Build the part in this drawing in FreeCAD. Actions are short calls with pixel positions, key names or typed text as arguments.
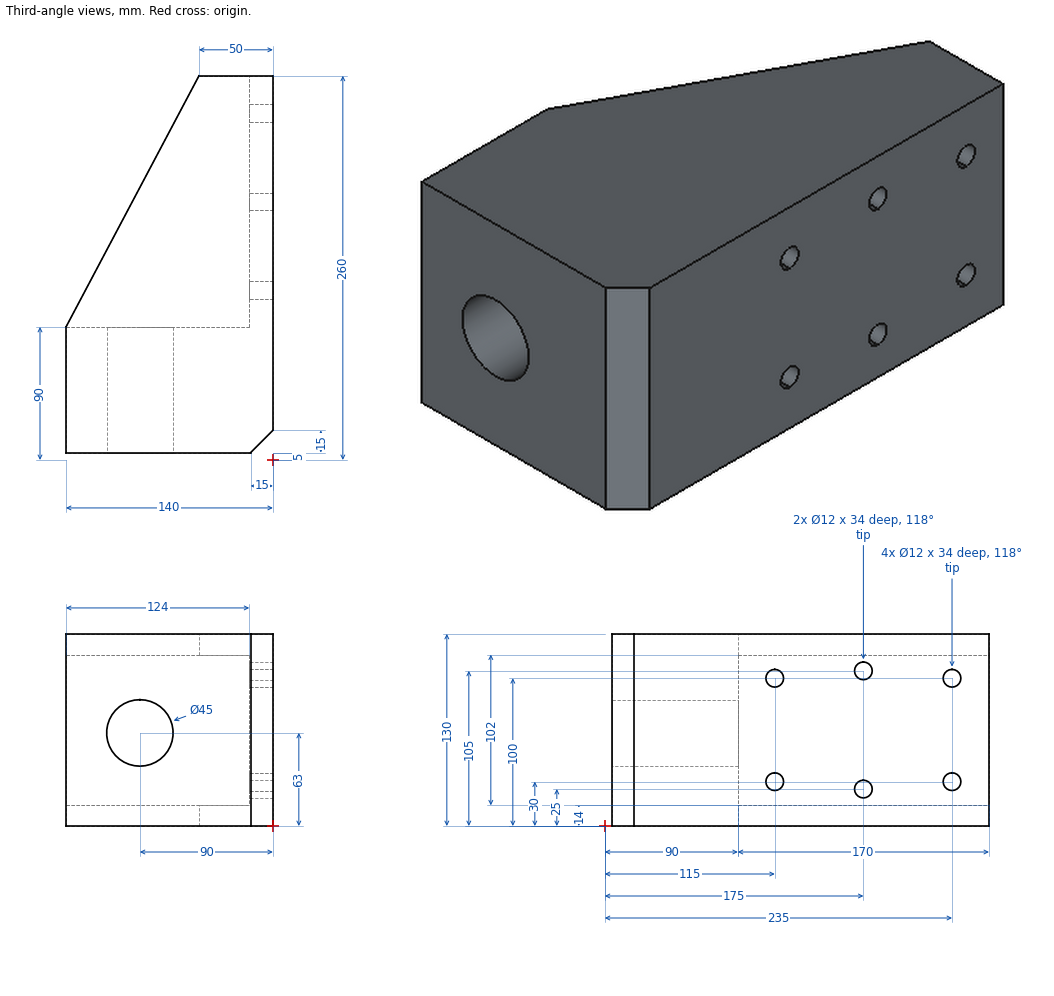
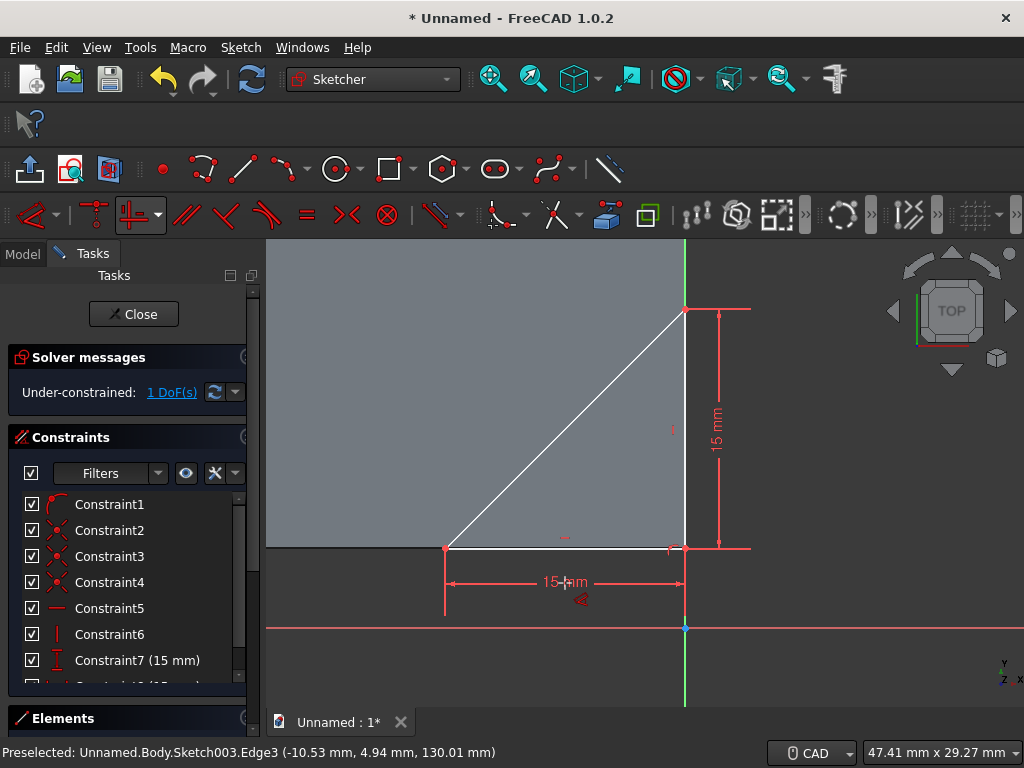
click(685, 549)
click(719, 589)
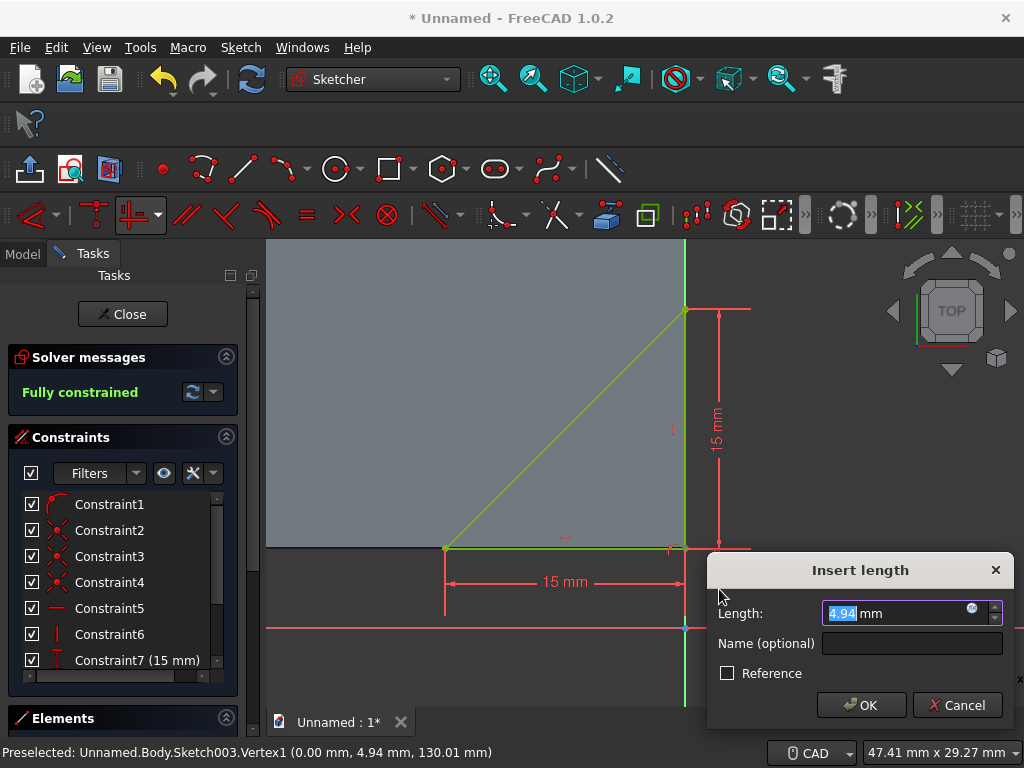
text(5)
key(Return)
key(Escape)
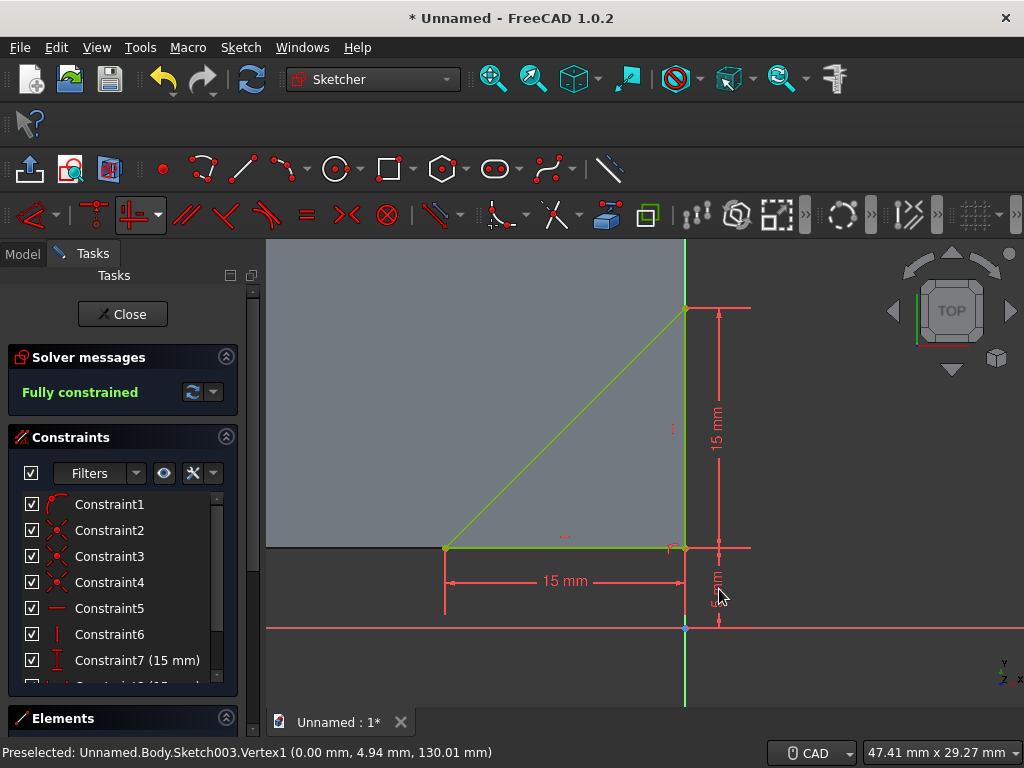
click(123, 314)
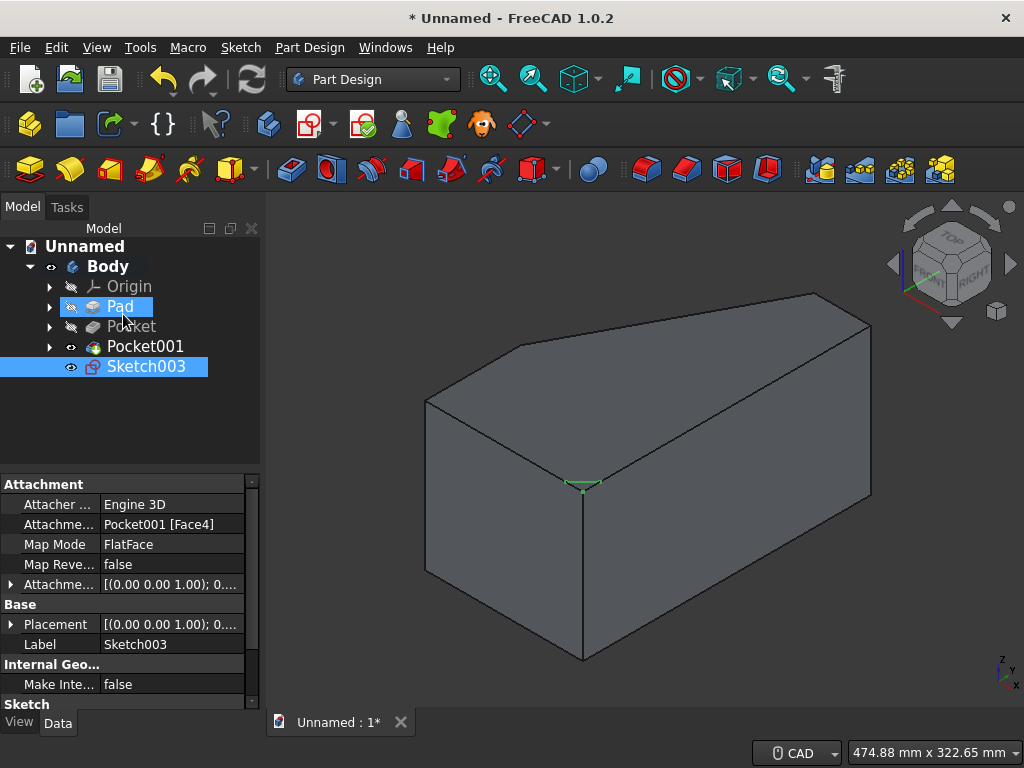
click(292, 170)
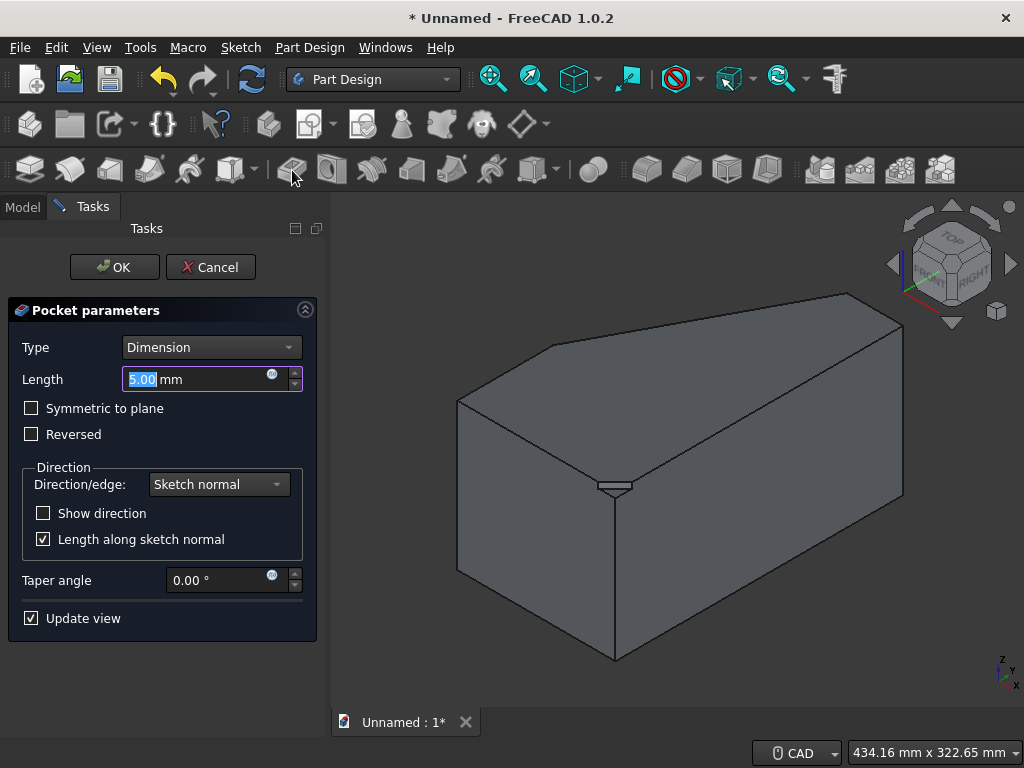
click(212, 348)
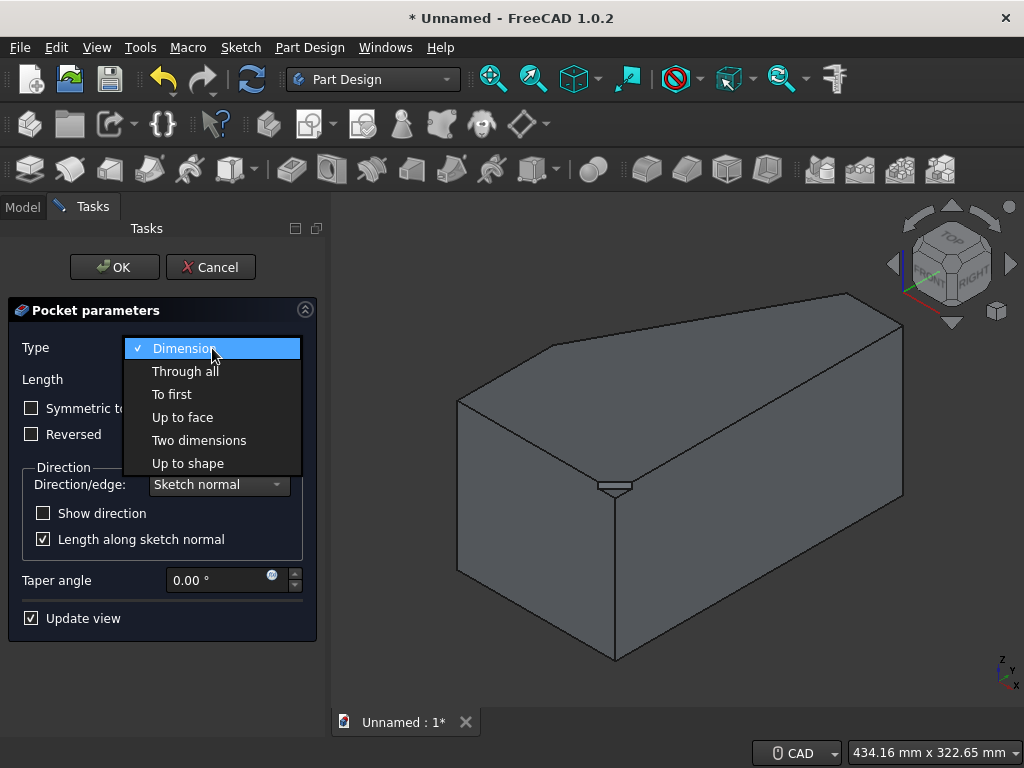
click(212, 372)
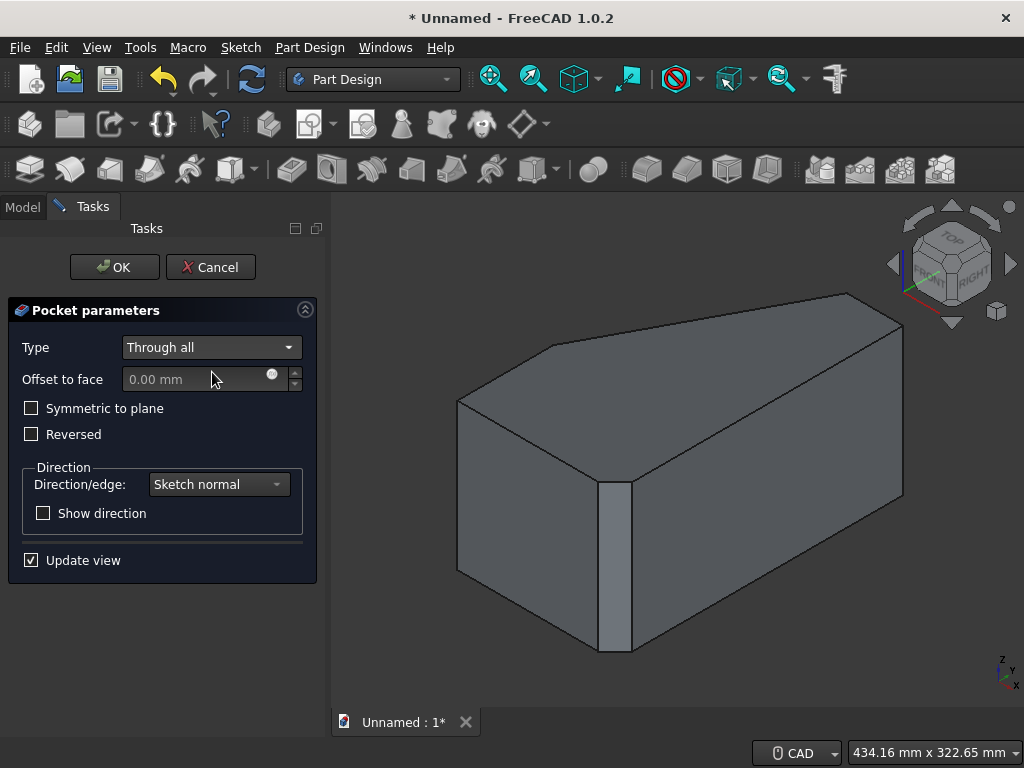
click(115, 267)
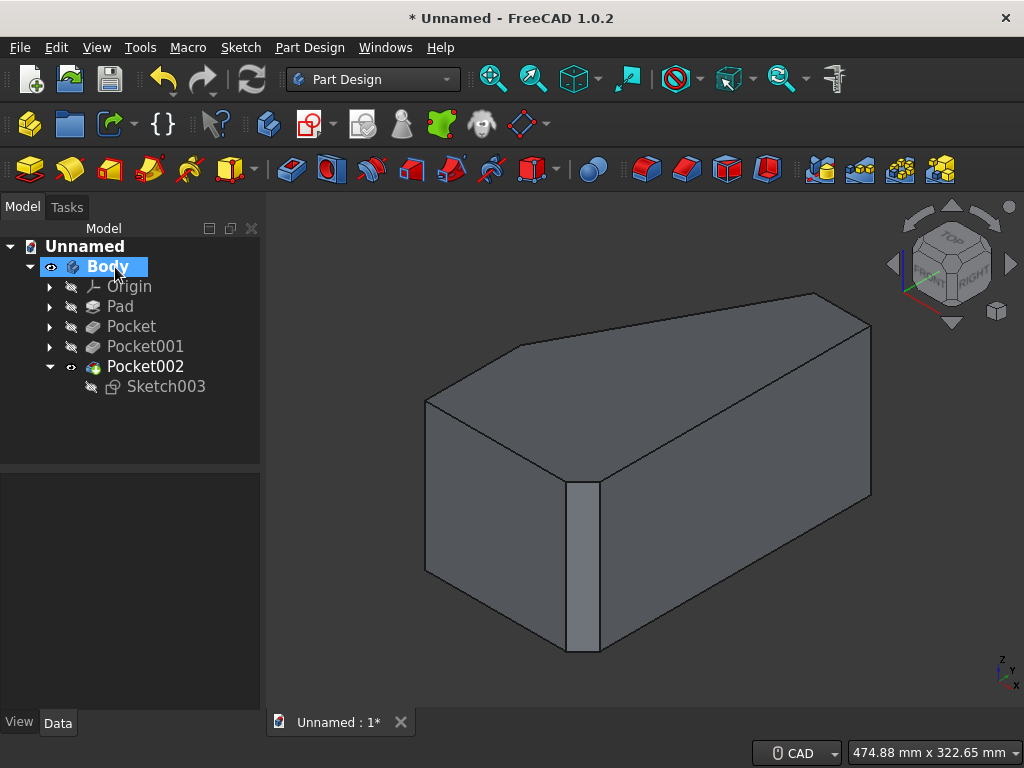
click(310, 124)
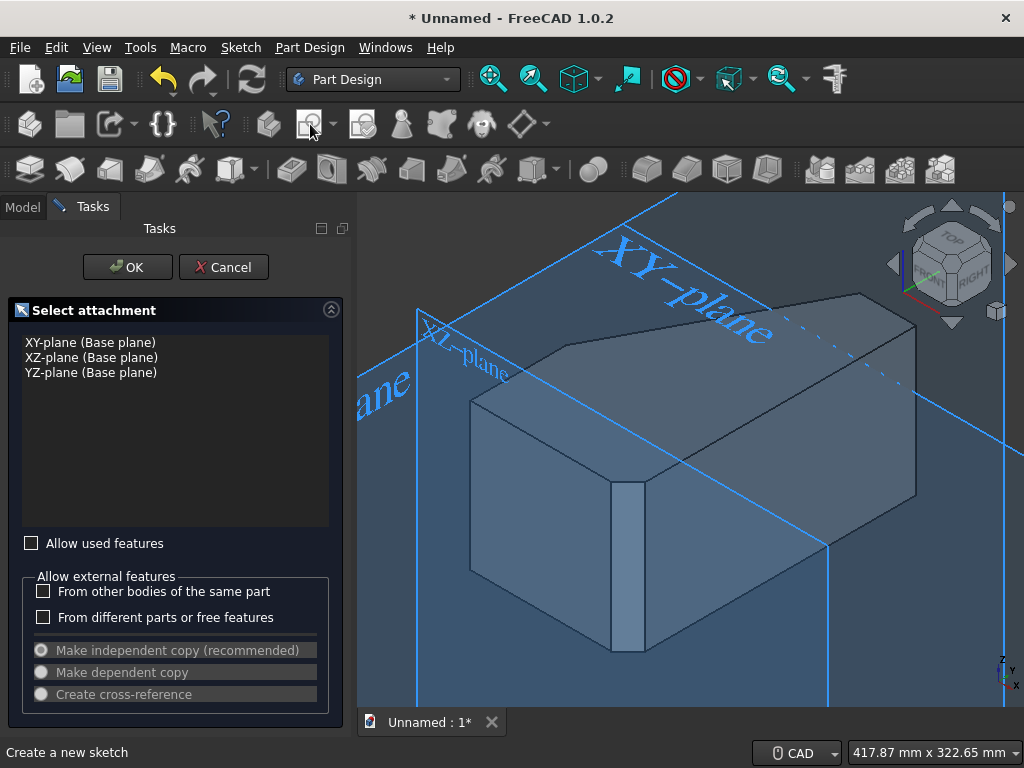
click(82, 372)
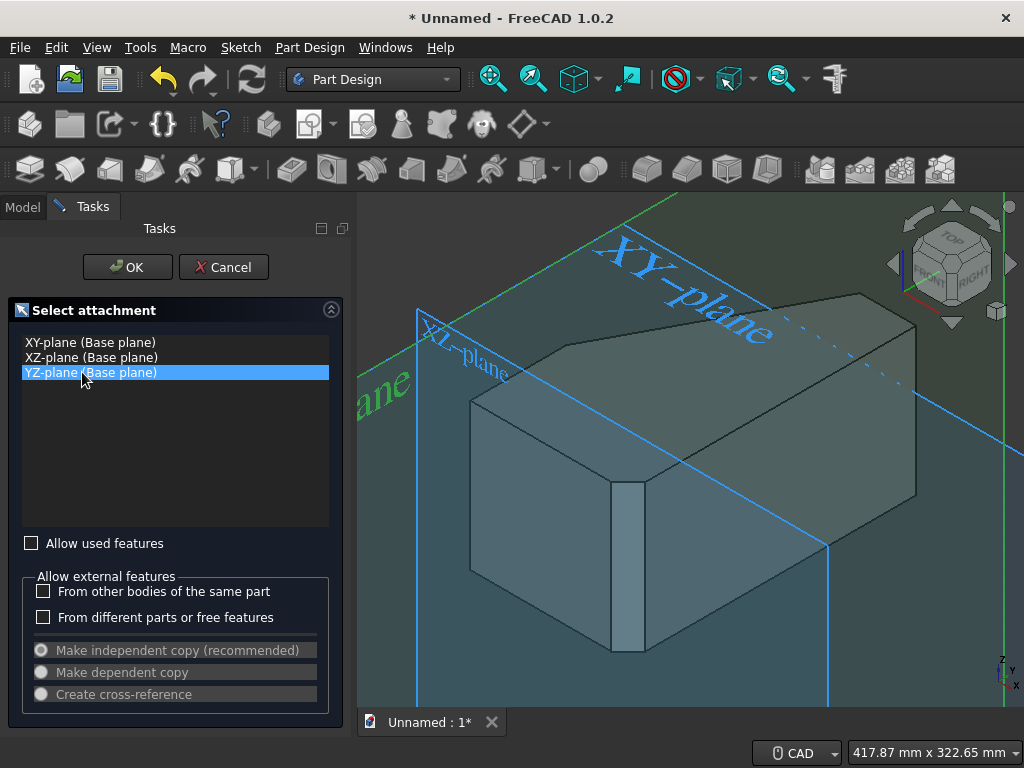
click(128, 267)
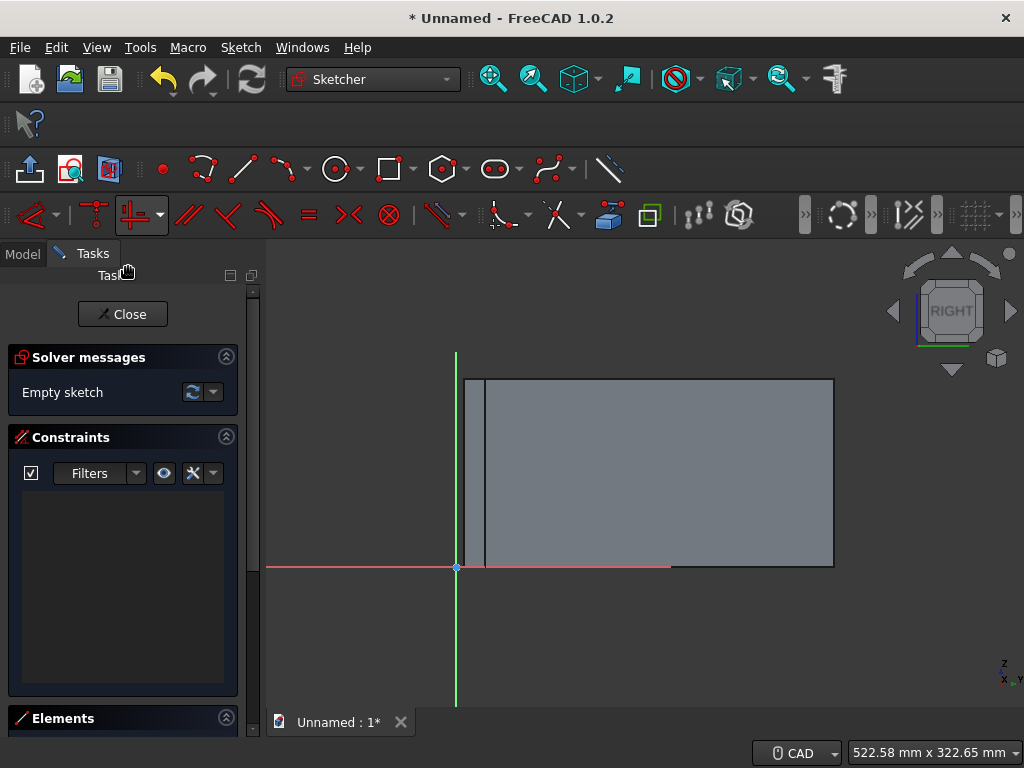
click(336, 170)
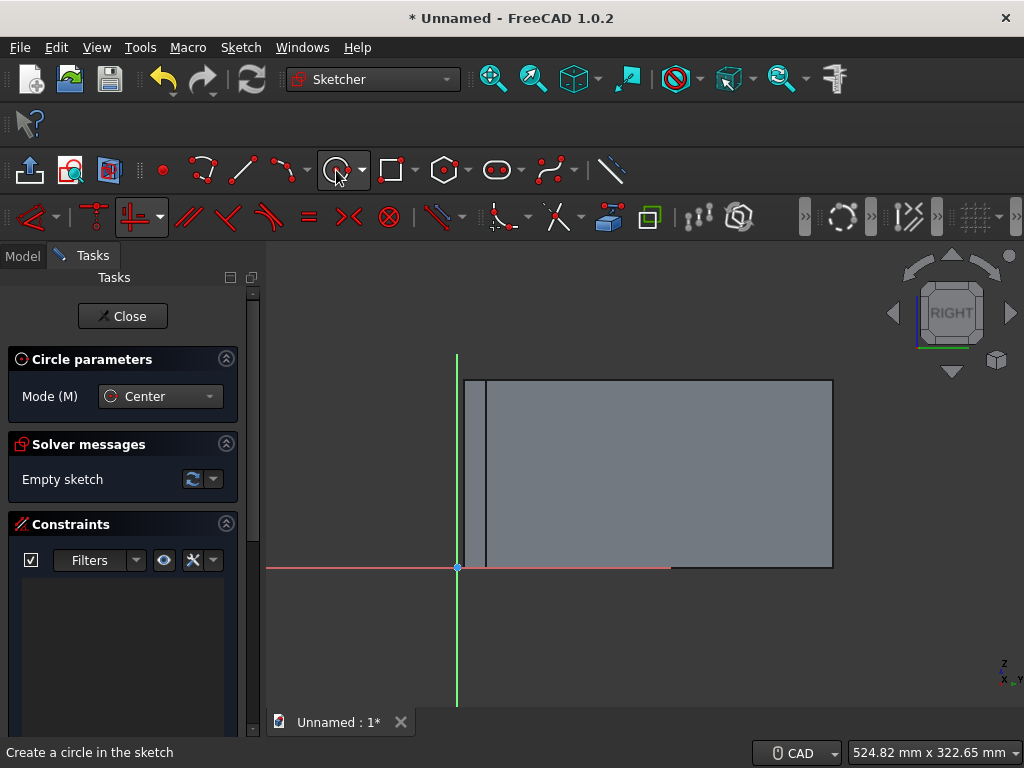
scroll(797, 423, up, 5)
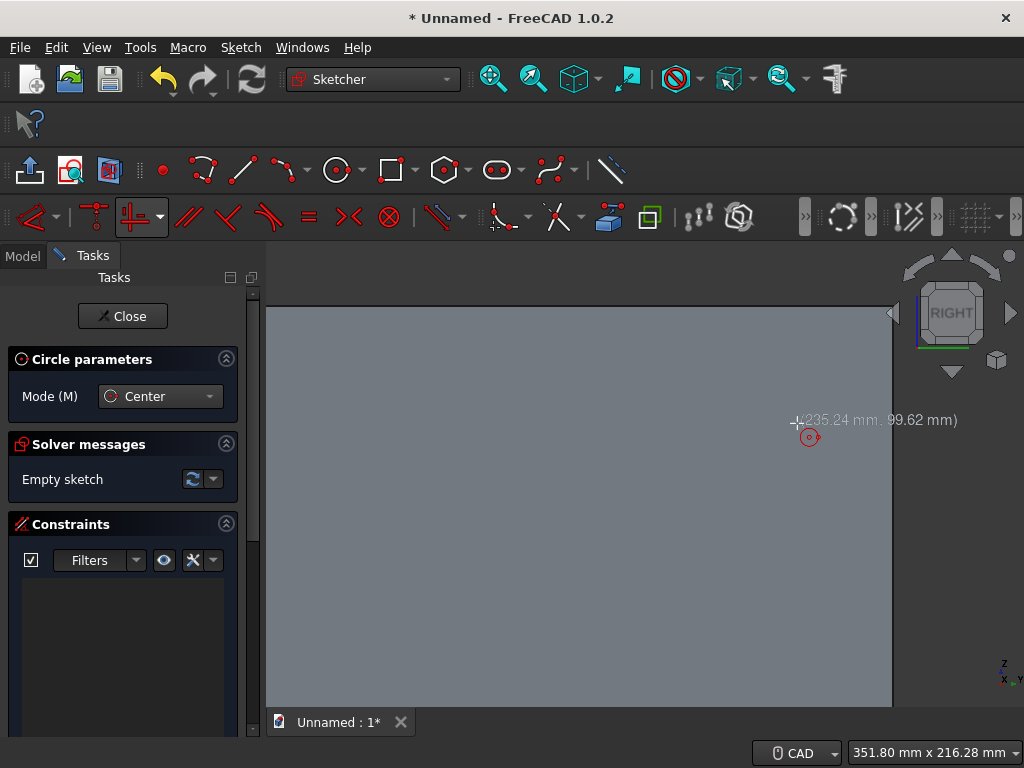
click(795, 424)
move(812, 407)